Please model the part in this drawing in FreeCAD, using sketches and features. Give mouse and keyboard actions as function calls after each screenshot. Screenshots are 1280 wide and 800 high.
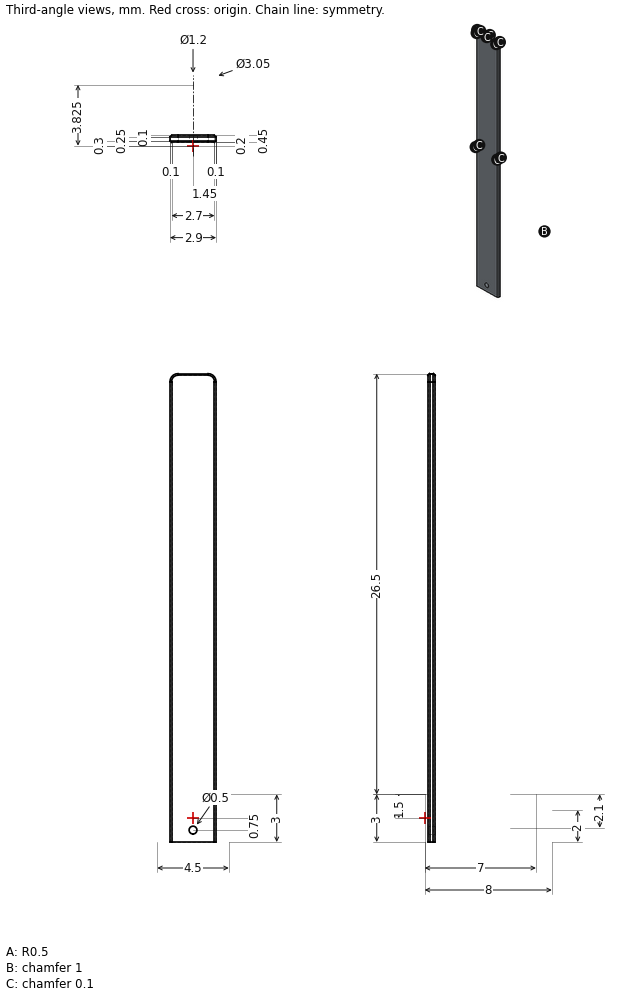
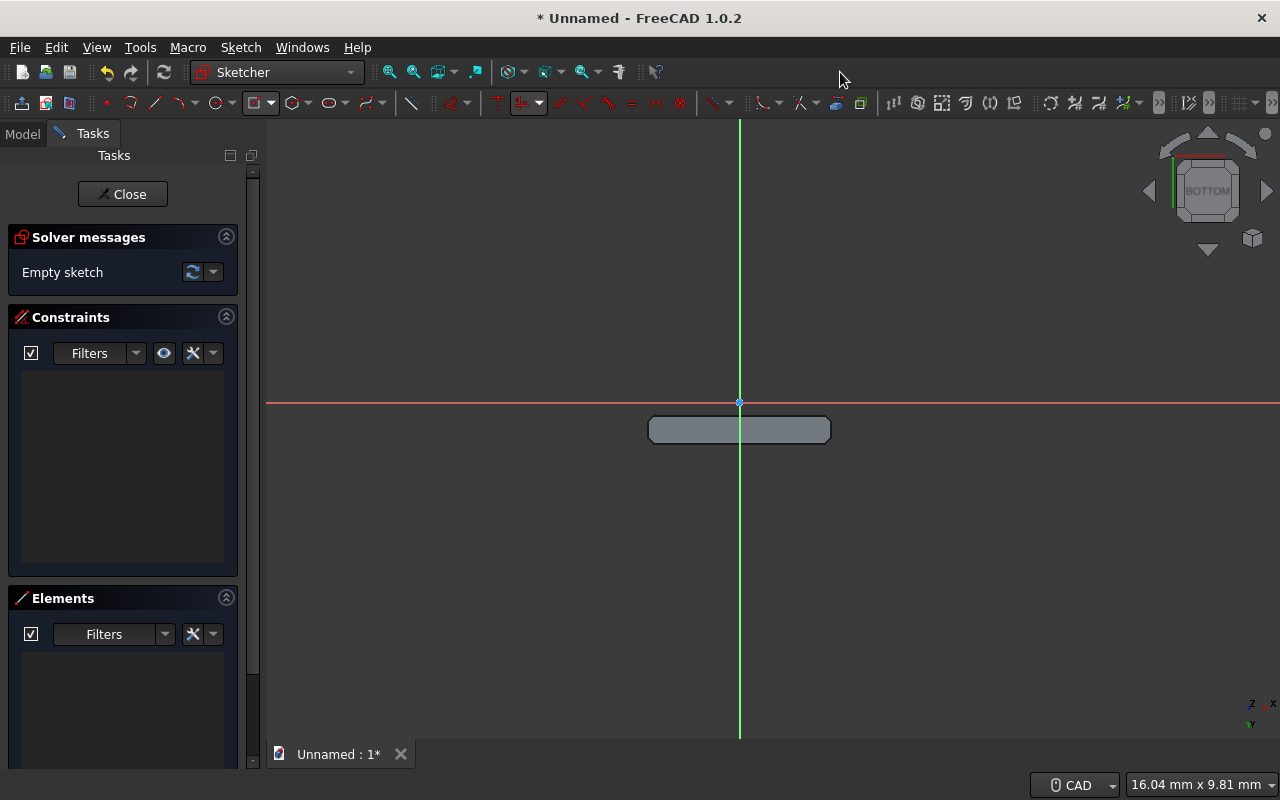
scroll(755, 421, up, 6)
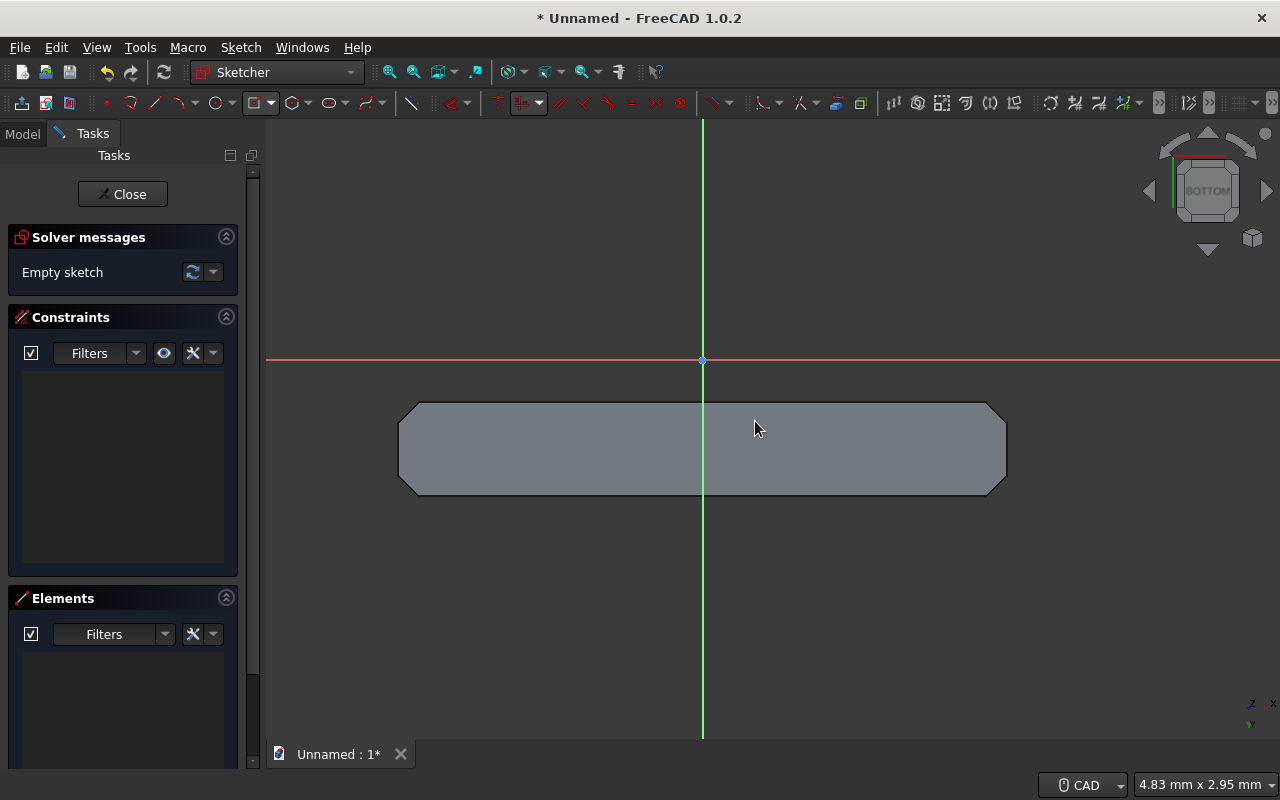
key(g)
key(m)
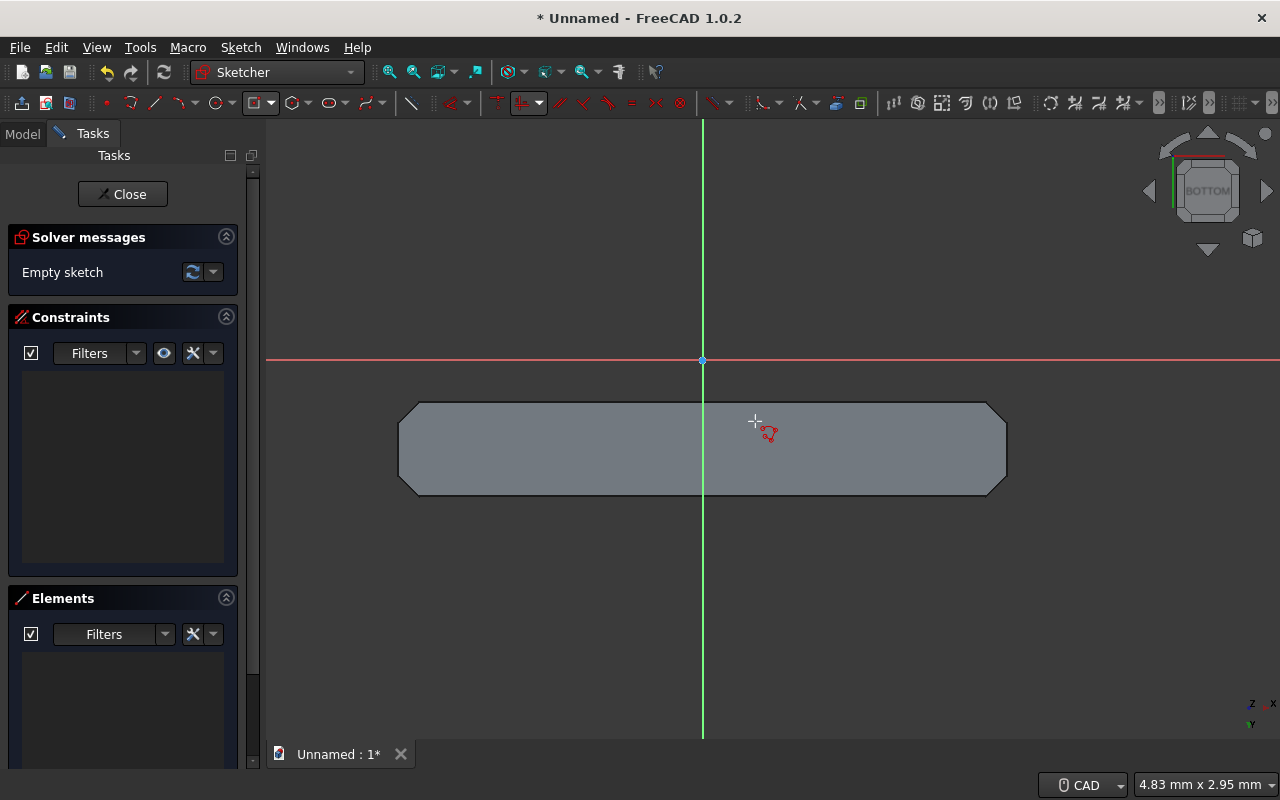
click(986, 402)
click(419, 402)
click(398, 423)
click(398, 476)
click(419, 496)
click(986, 496)
click(1007, 476)
click(1007, 423)
click(986, 403)
key(Escape)
key(Escape)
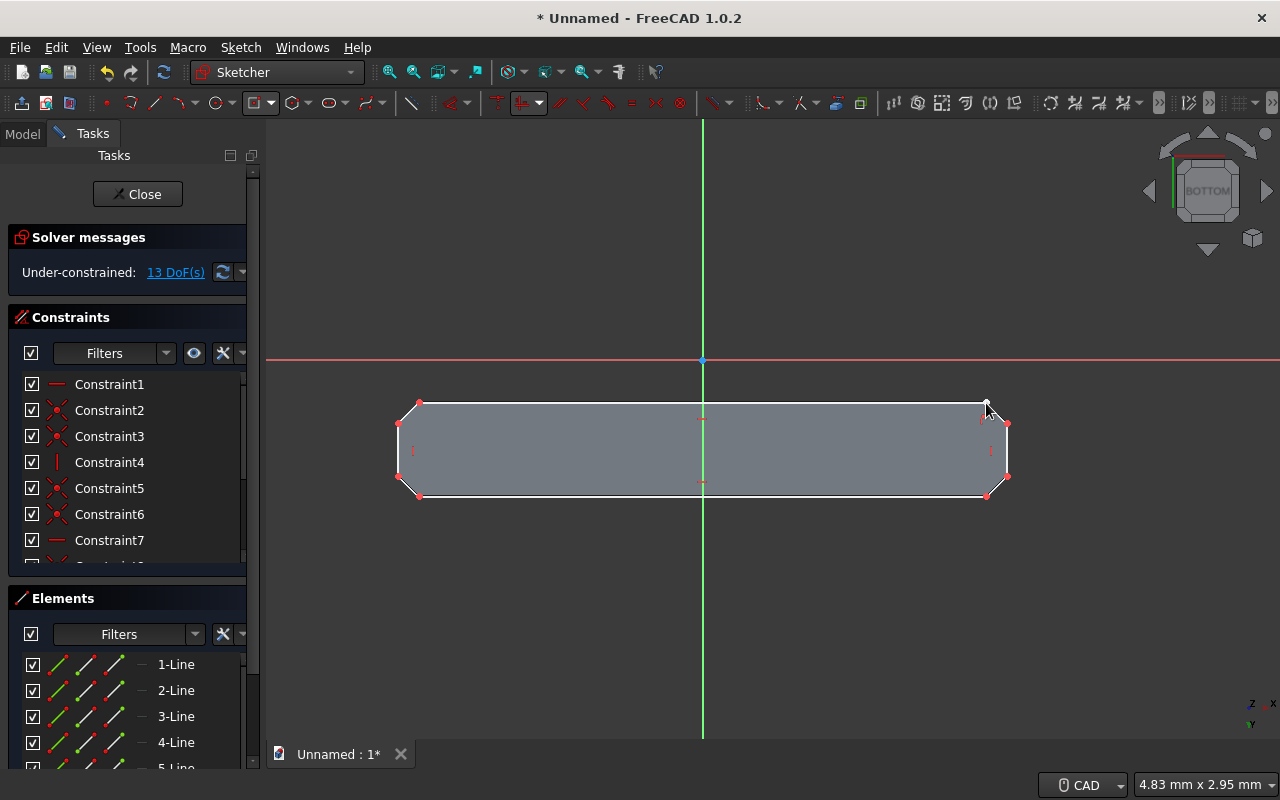
click(398, 477)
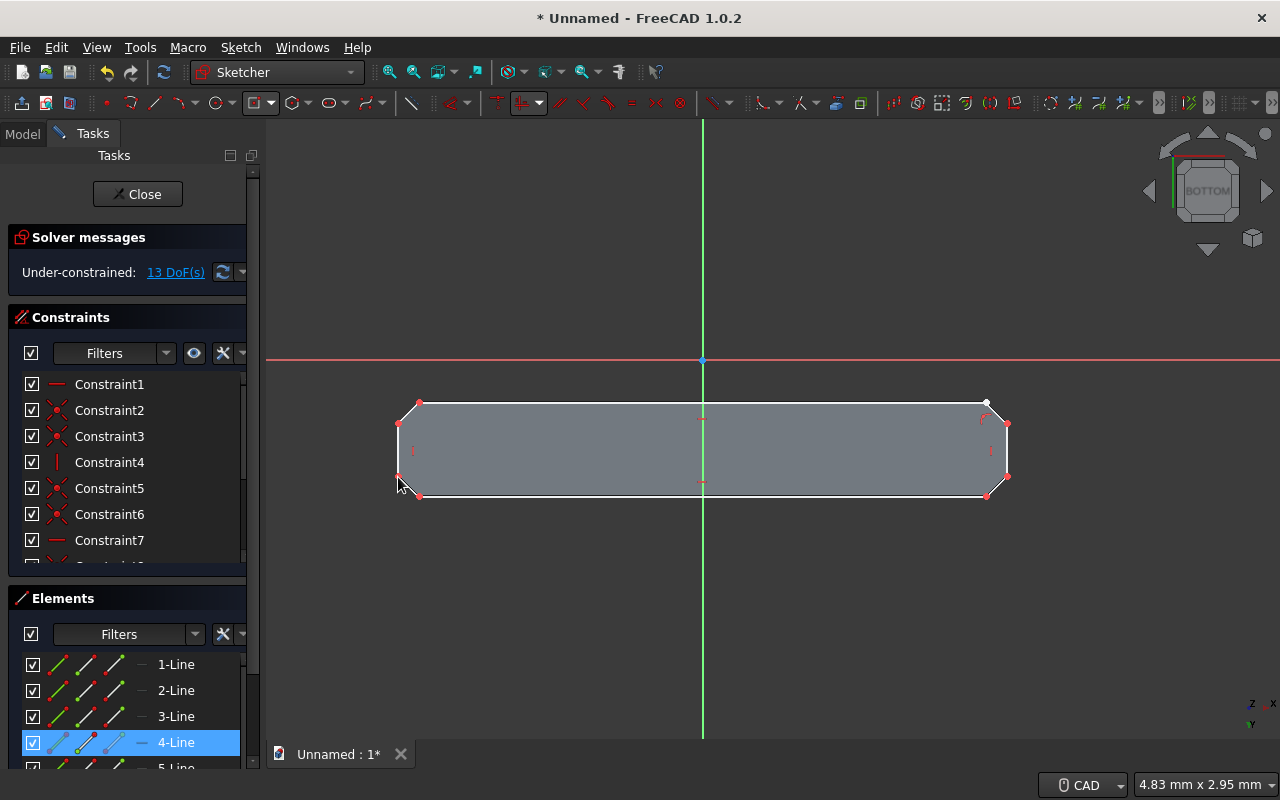
click(1007, 477)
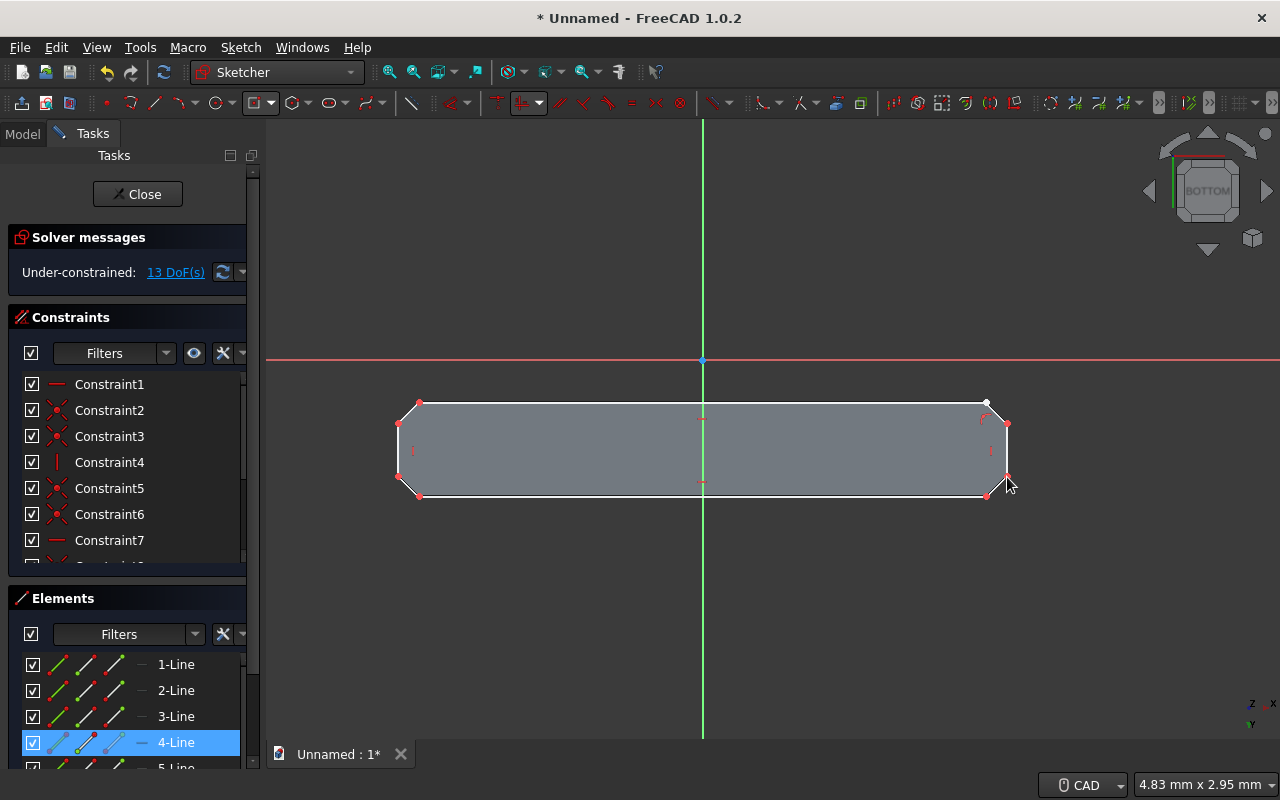
click(703, 671)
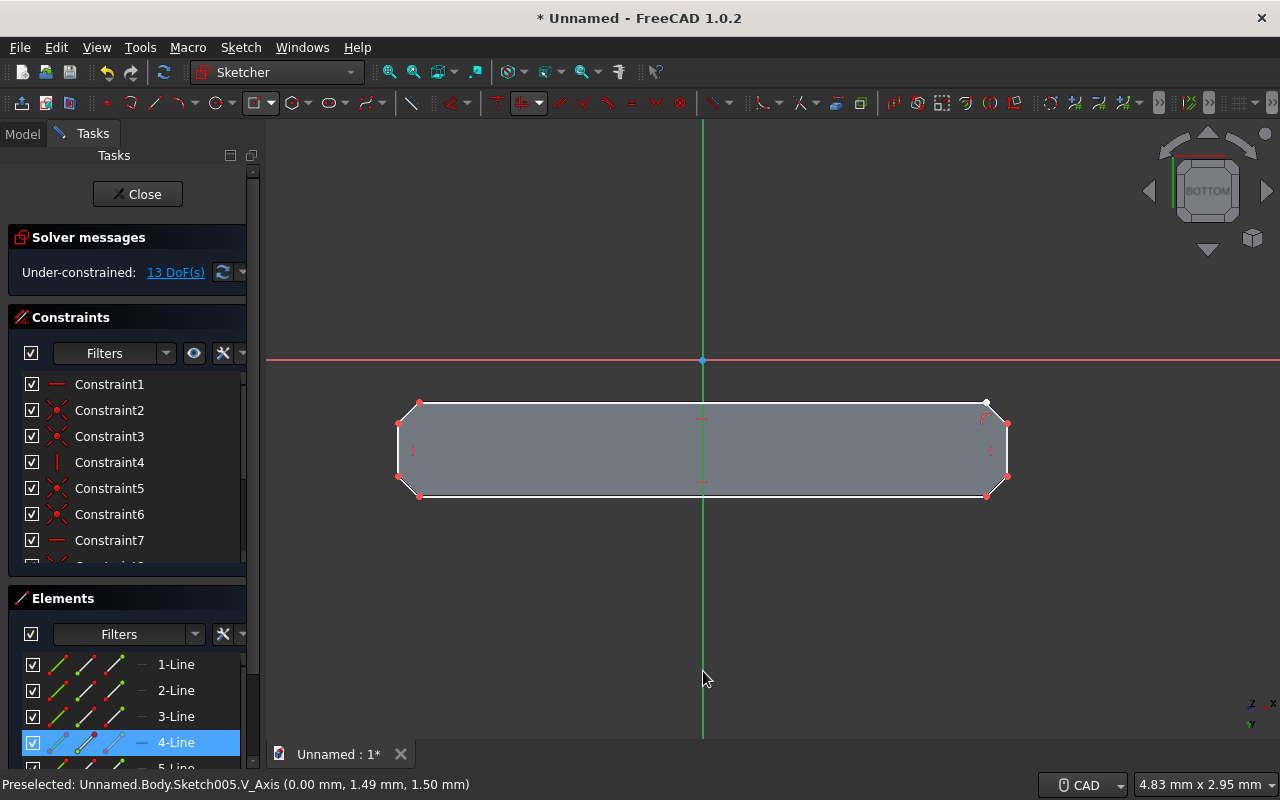
key(s)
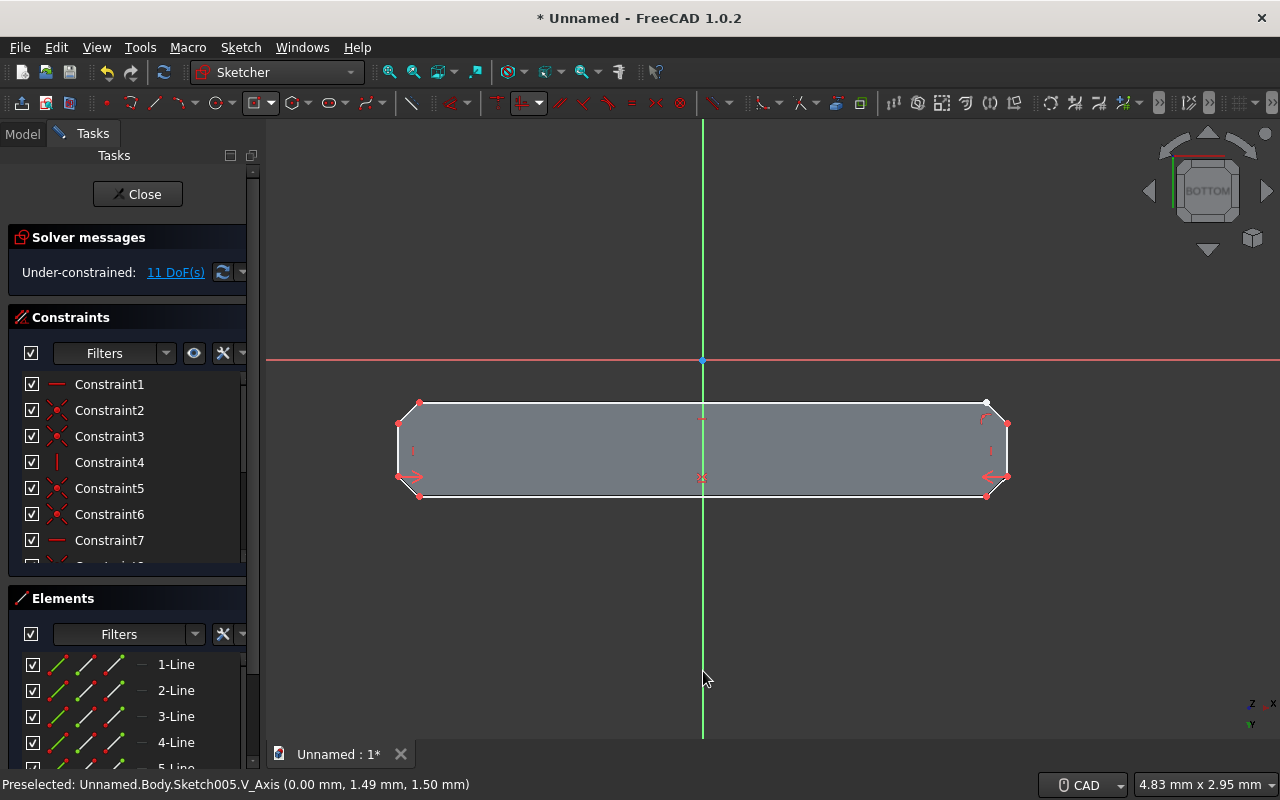
click(450, 104)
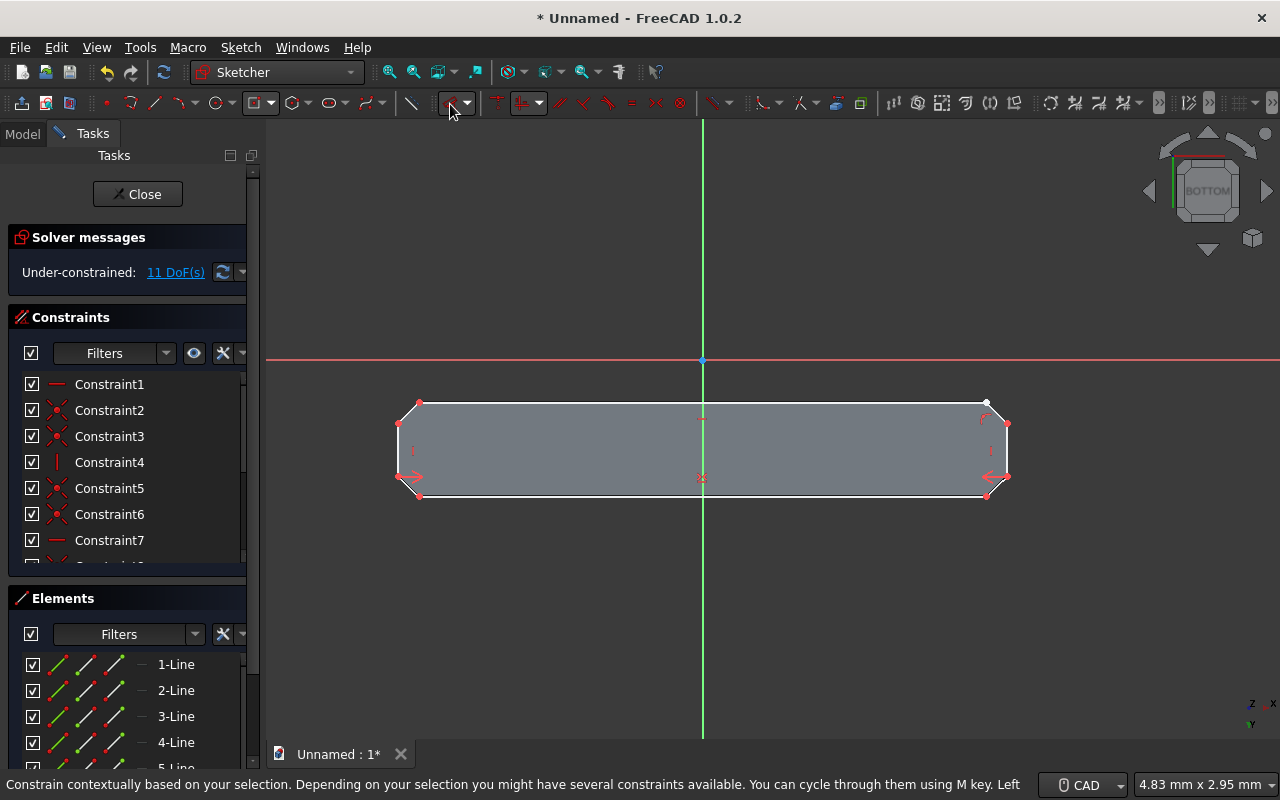
click(816, 403)
click(572, 437)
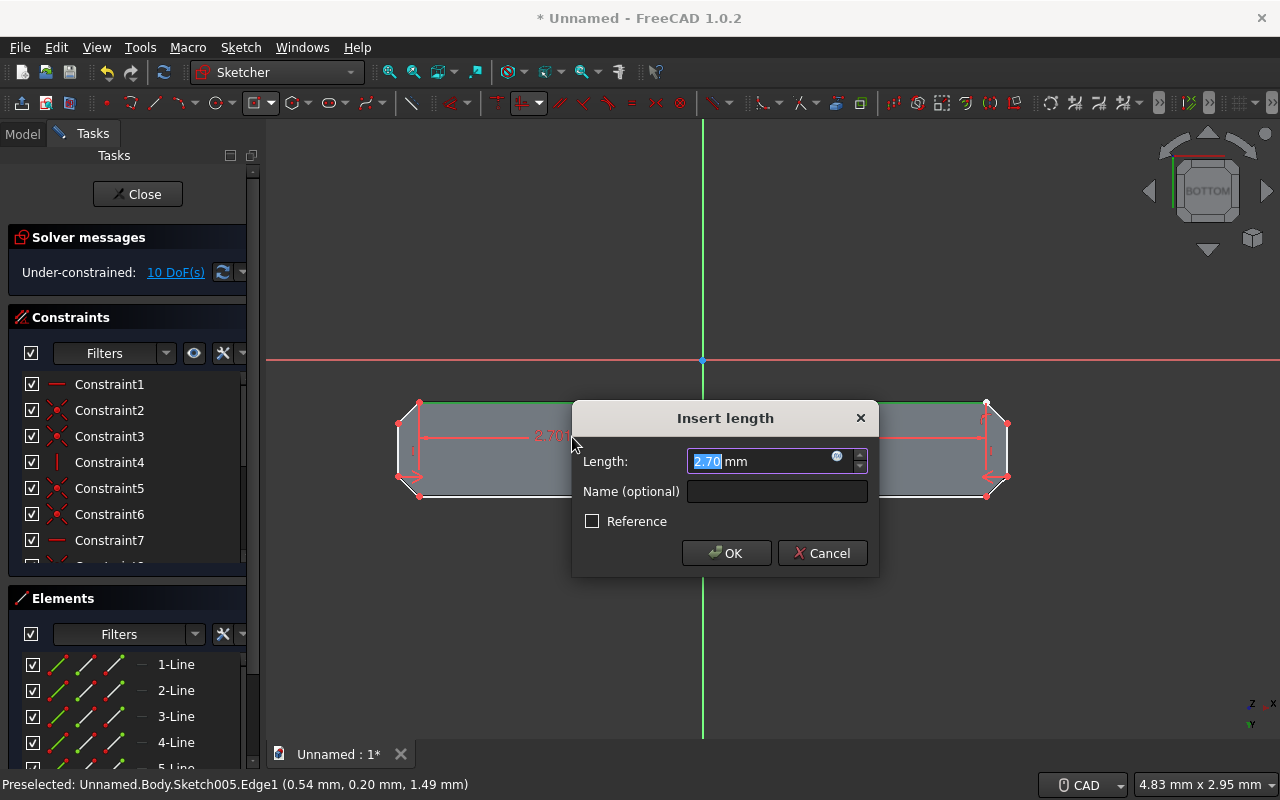
text(2.7)
key(Return)